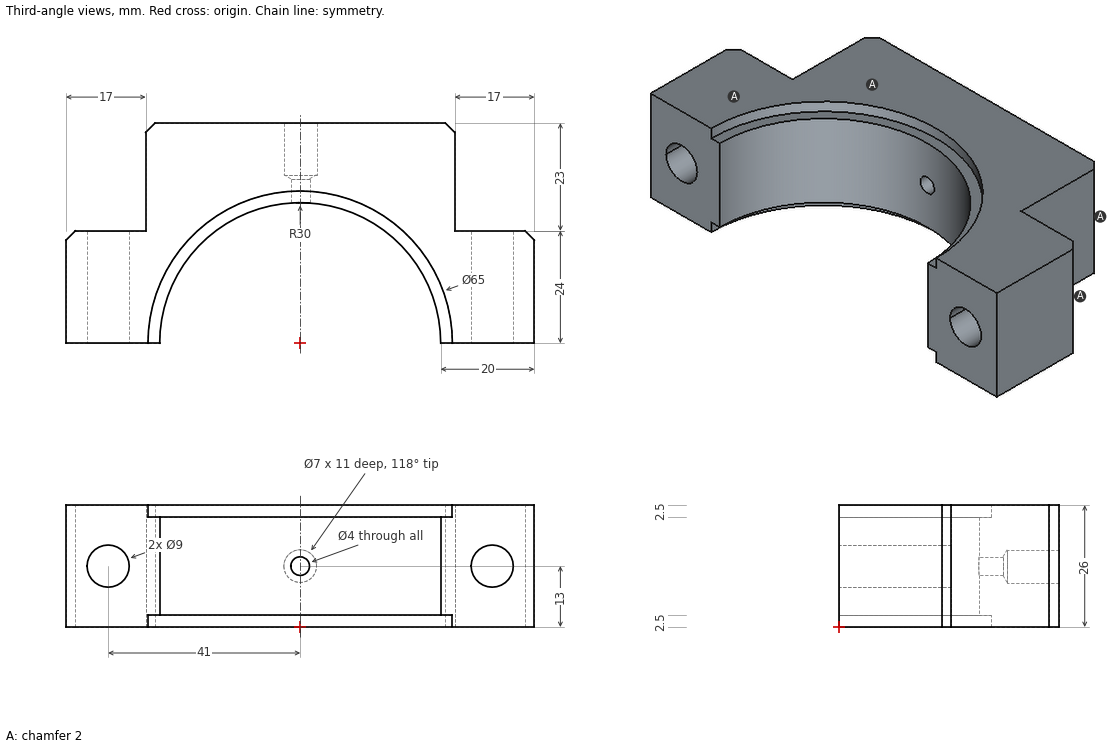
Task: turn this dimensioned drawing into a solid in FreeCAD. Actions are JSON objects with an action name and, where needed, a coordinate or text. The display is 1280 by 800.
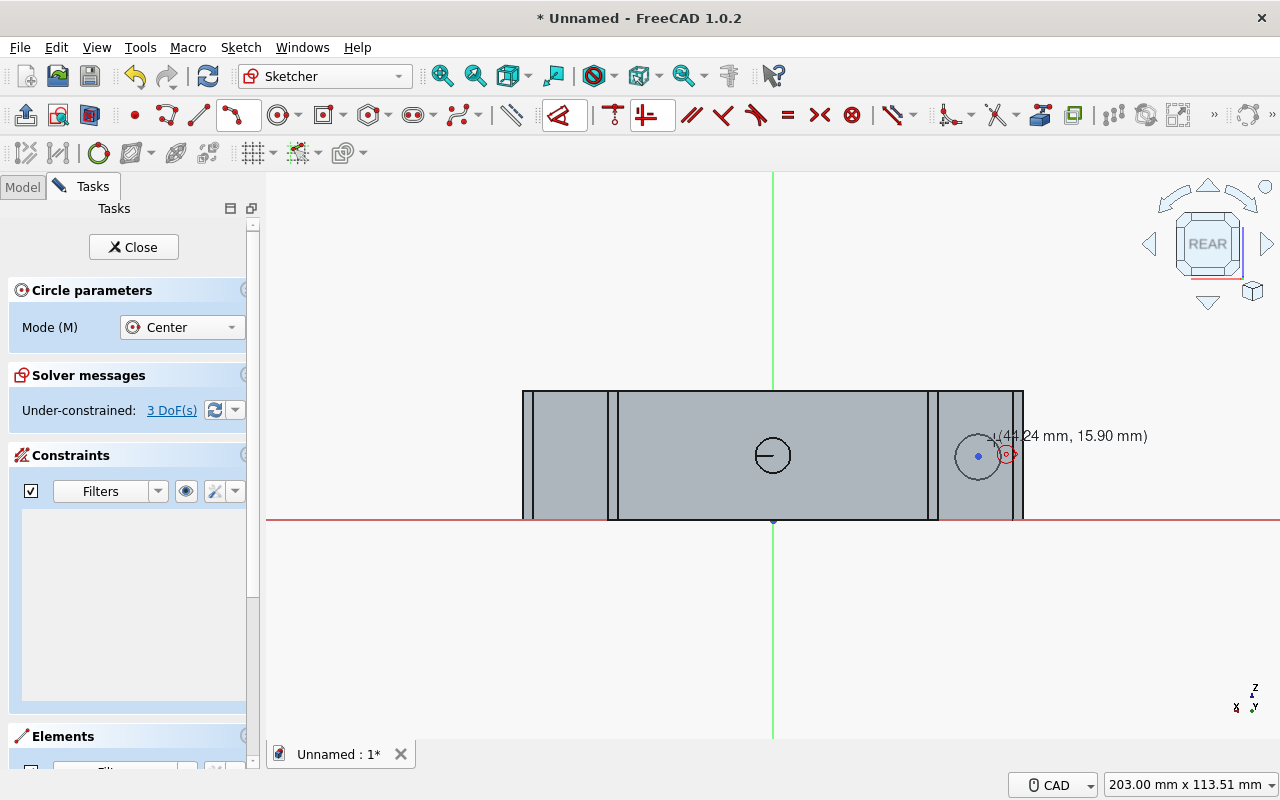
{"action": "left_click", "coordinate": [568, 456]}
{"action": "left_click", "coordinate": [584, 440]}
{"action": "key", "text": "Escape"}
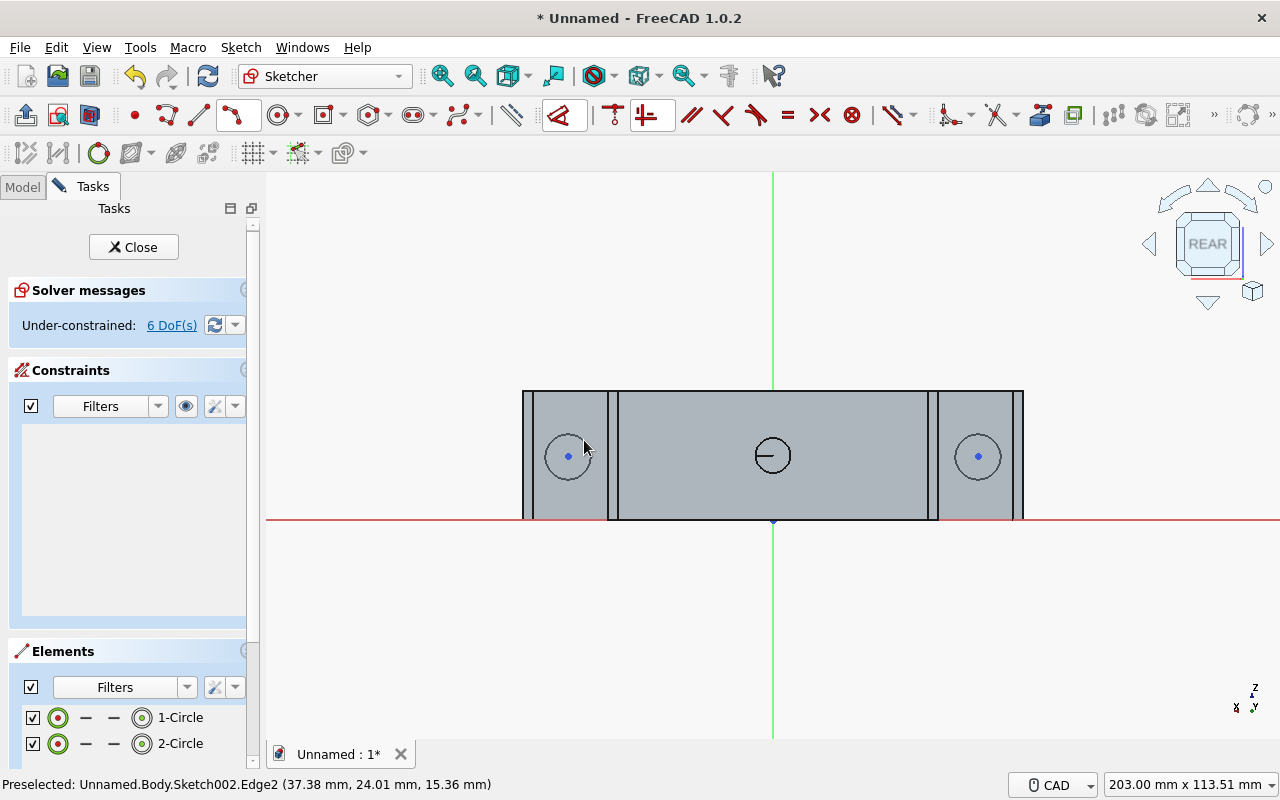
{"action": "left_click", "coordinate": [994, 441]}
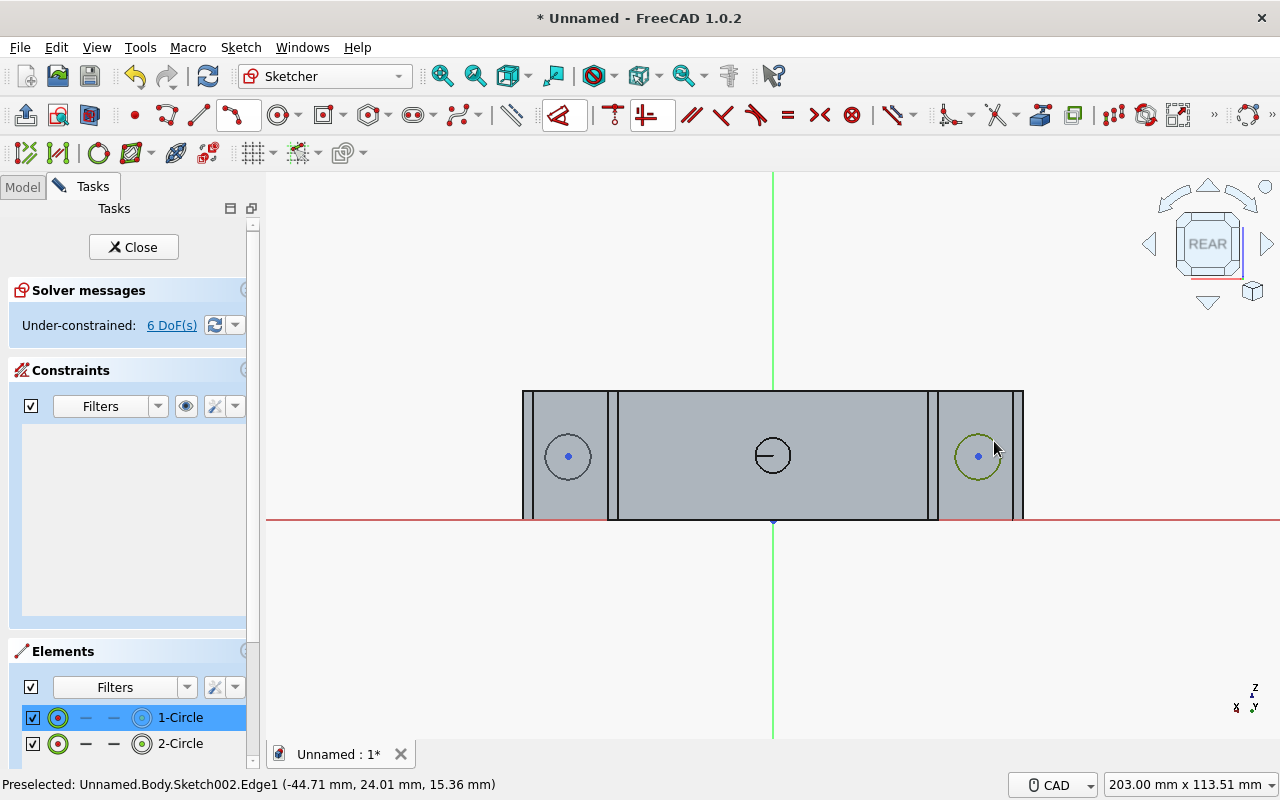
{"action": "left_click", "coordinate": [584, 441]}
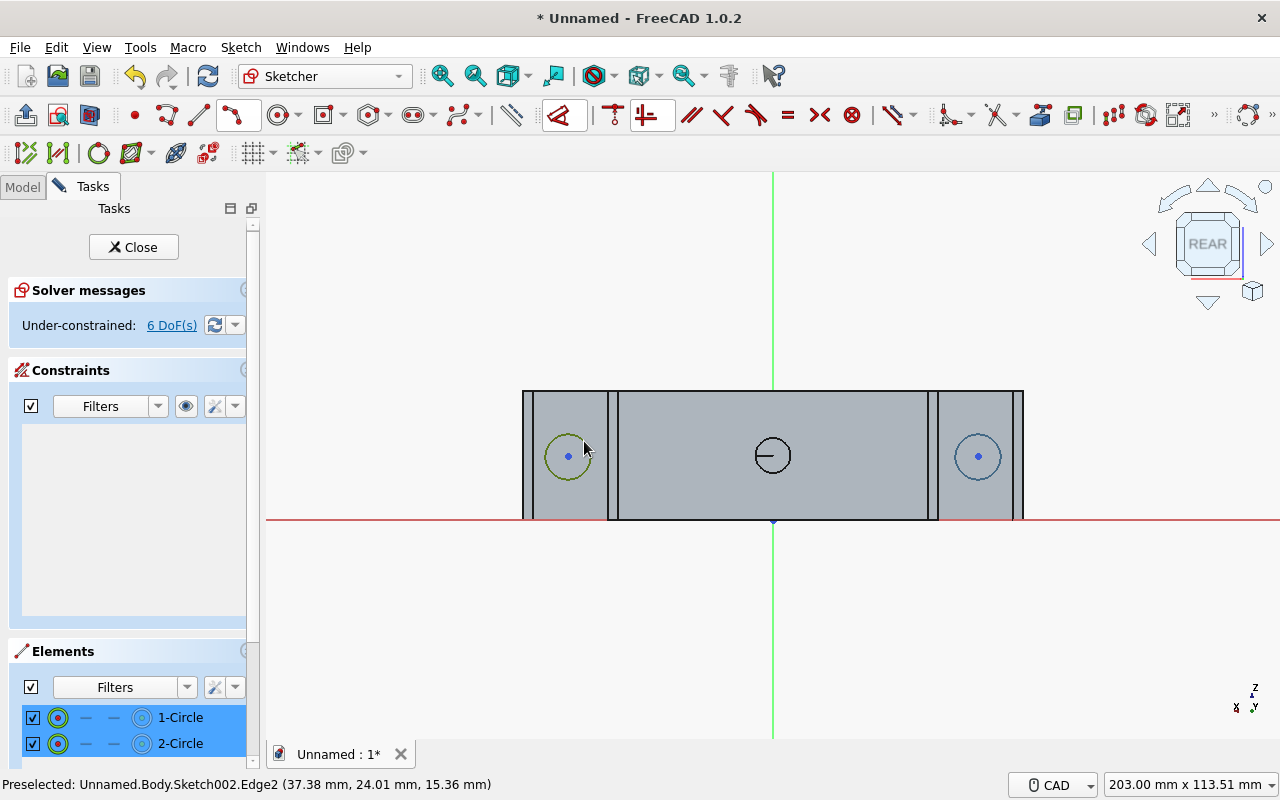
{"action": "left_click", "coordinate": [788, 116]}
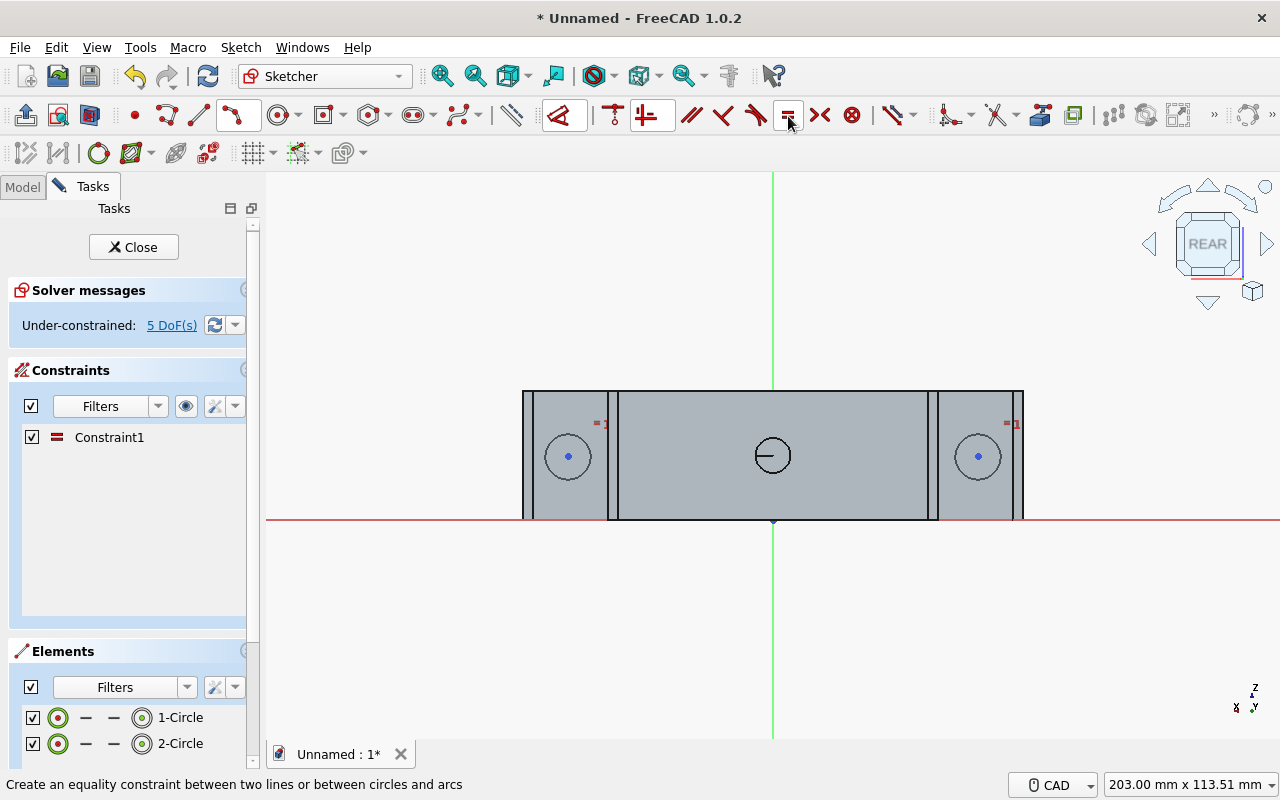
{"action": "left_click", "coordinate": [978, 457]}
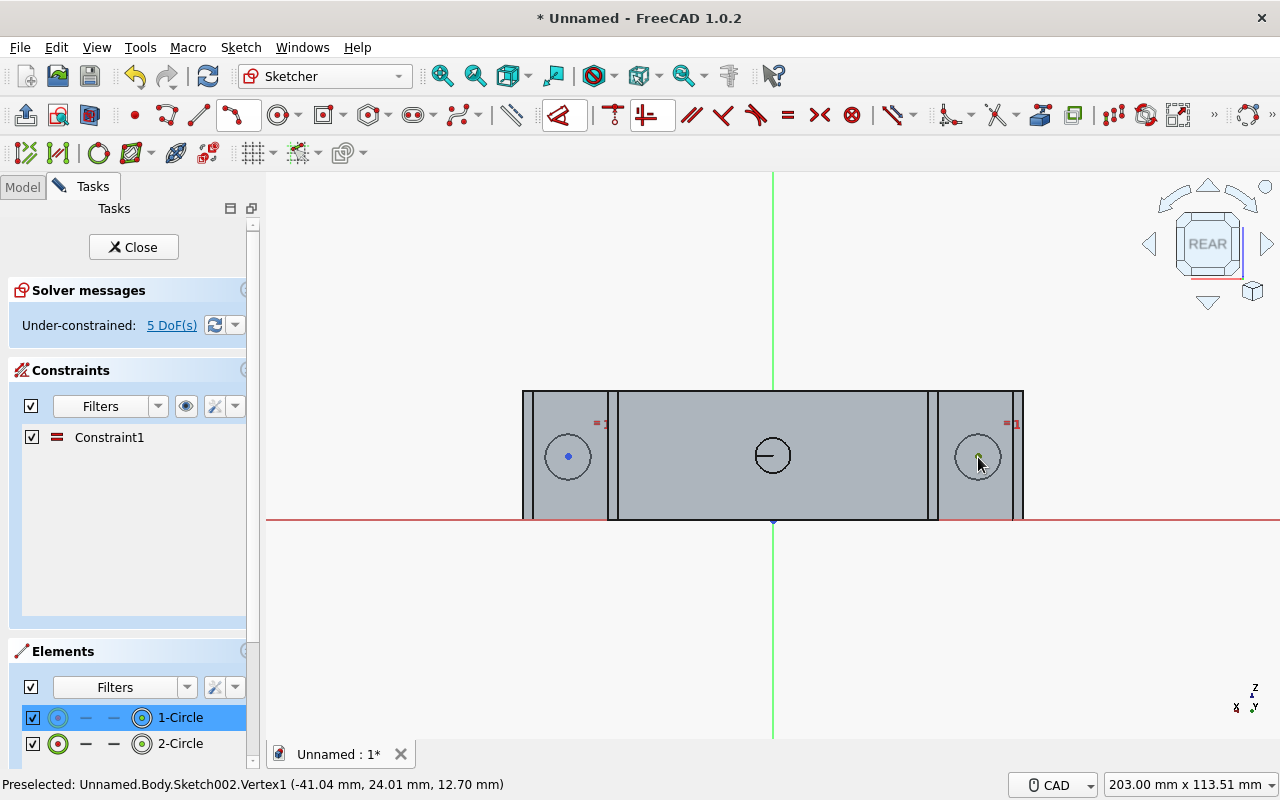
{"action": "left_click", "coordinate": [568, 457]}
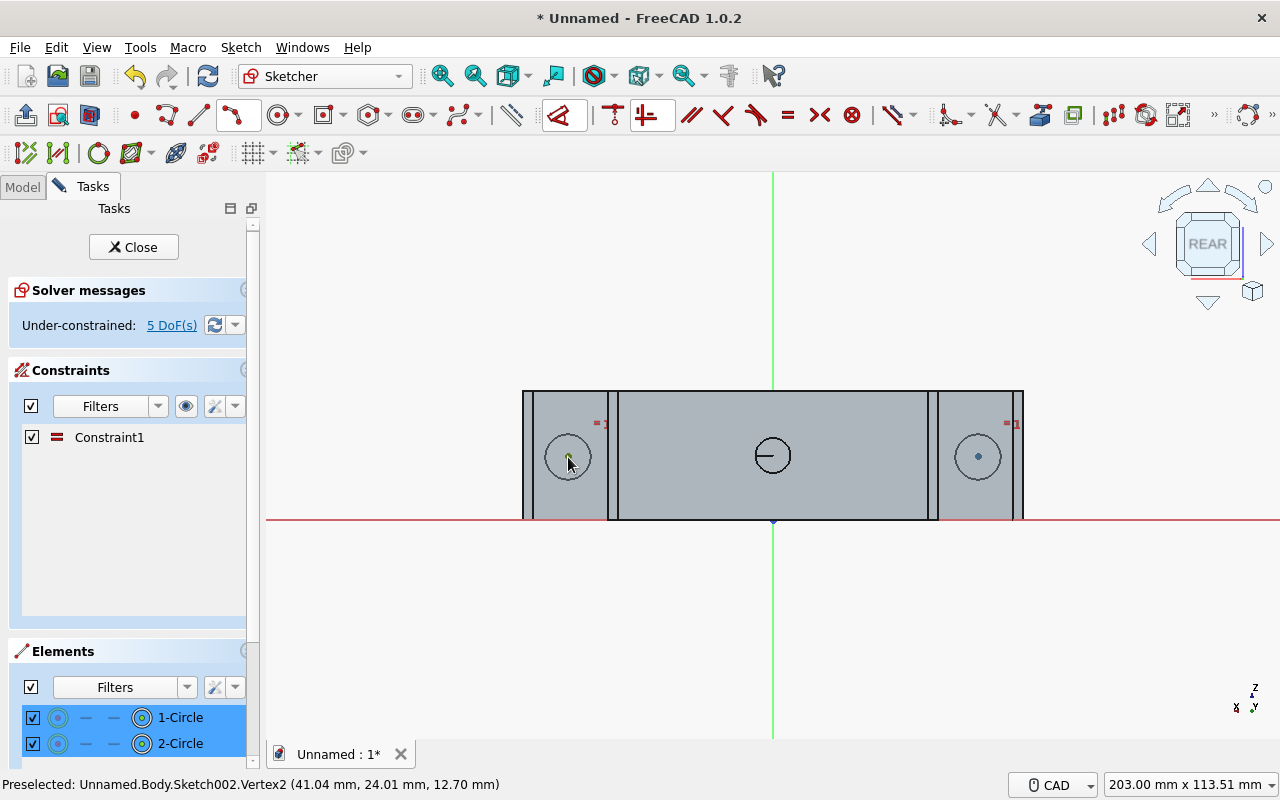
{"action": "left_click", "coordinate": [773, 674]}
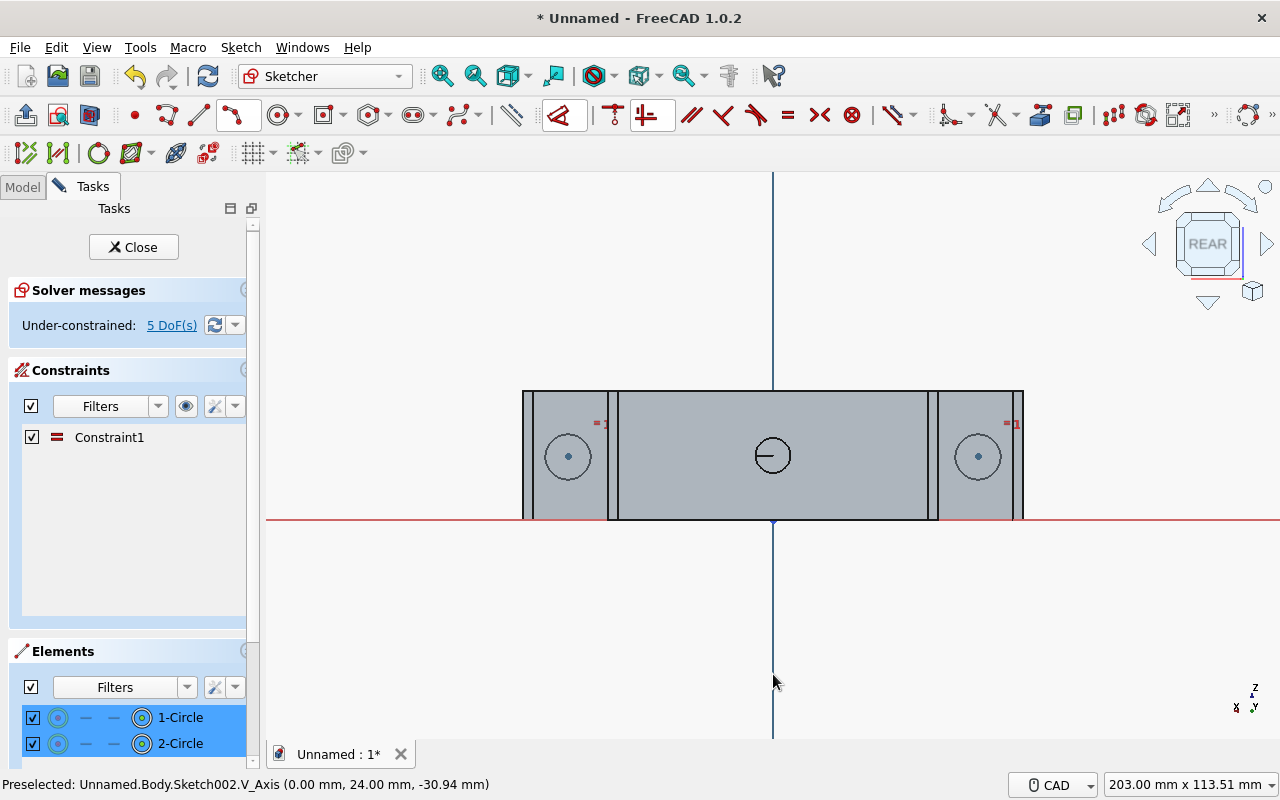
{"action": "key", "text": "s"}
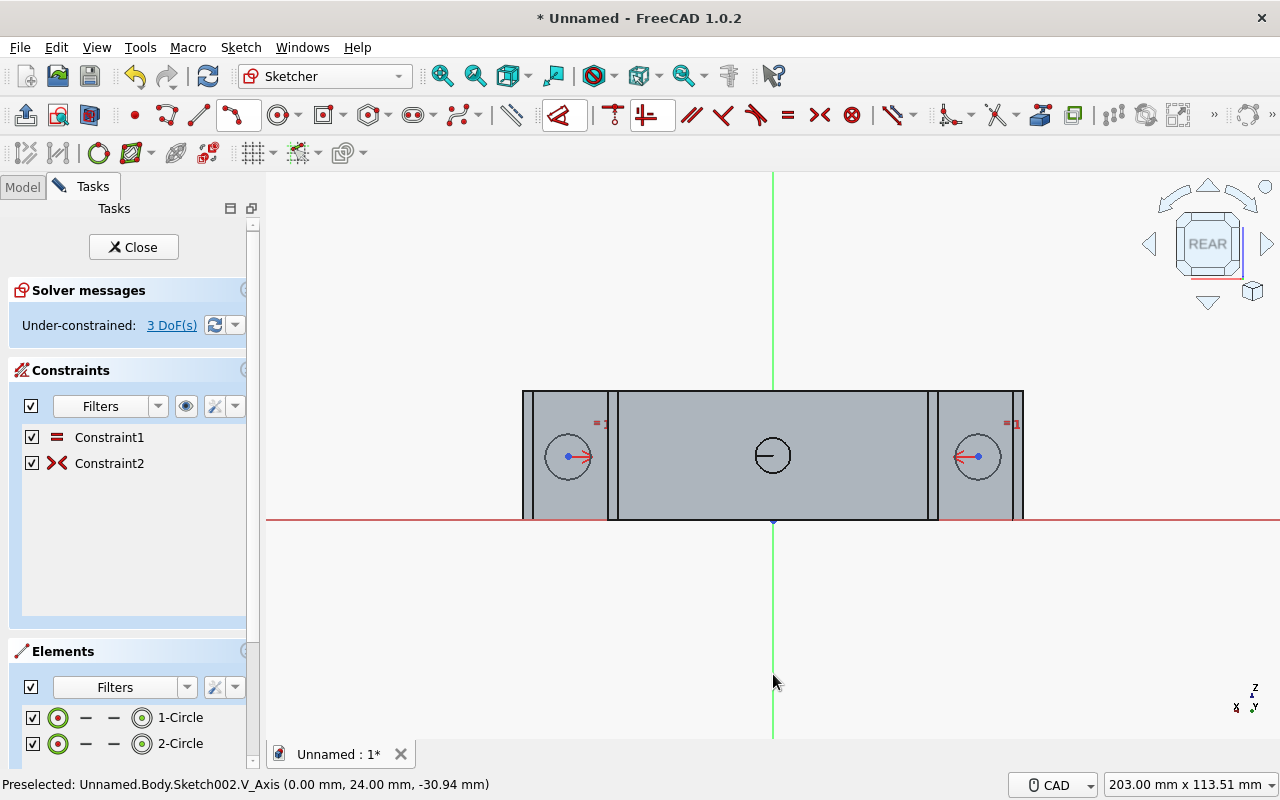
{"action": "left_click", "coordinate": [994, 441]}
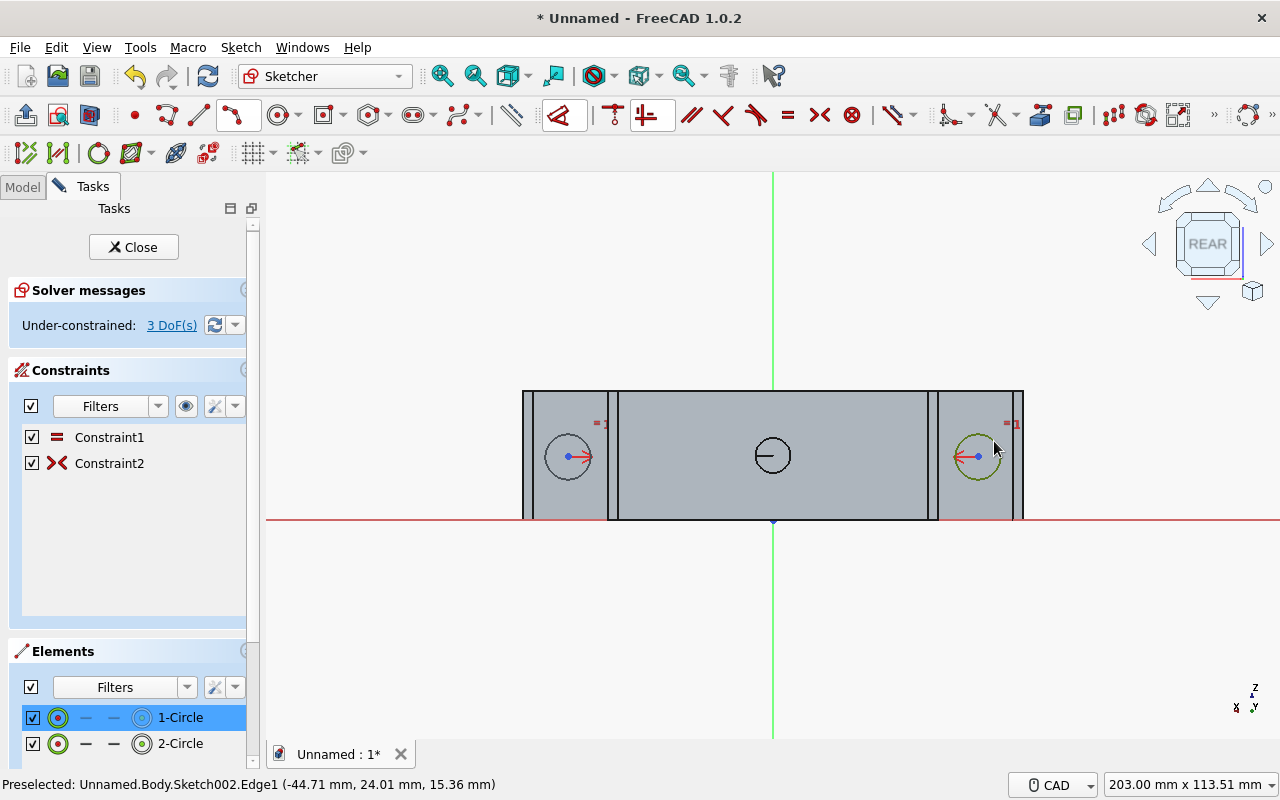
{"action": "key", "text": "k o"}